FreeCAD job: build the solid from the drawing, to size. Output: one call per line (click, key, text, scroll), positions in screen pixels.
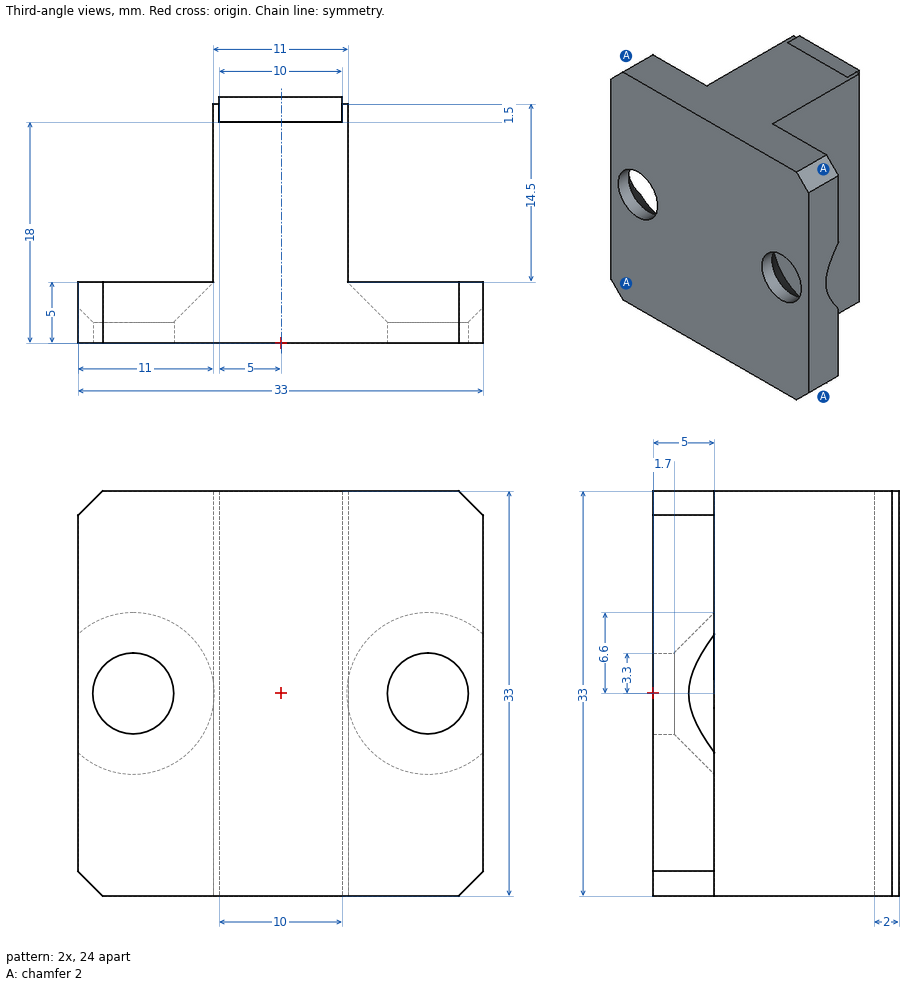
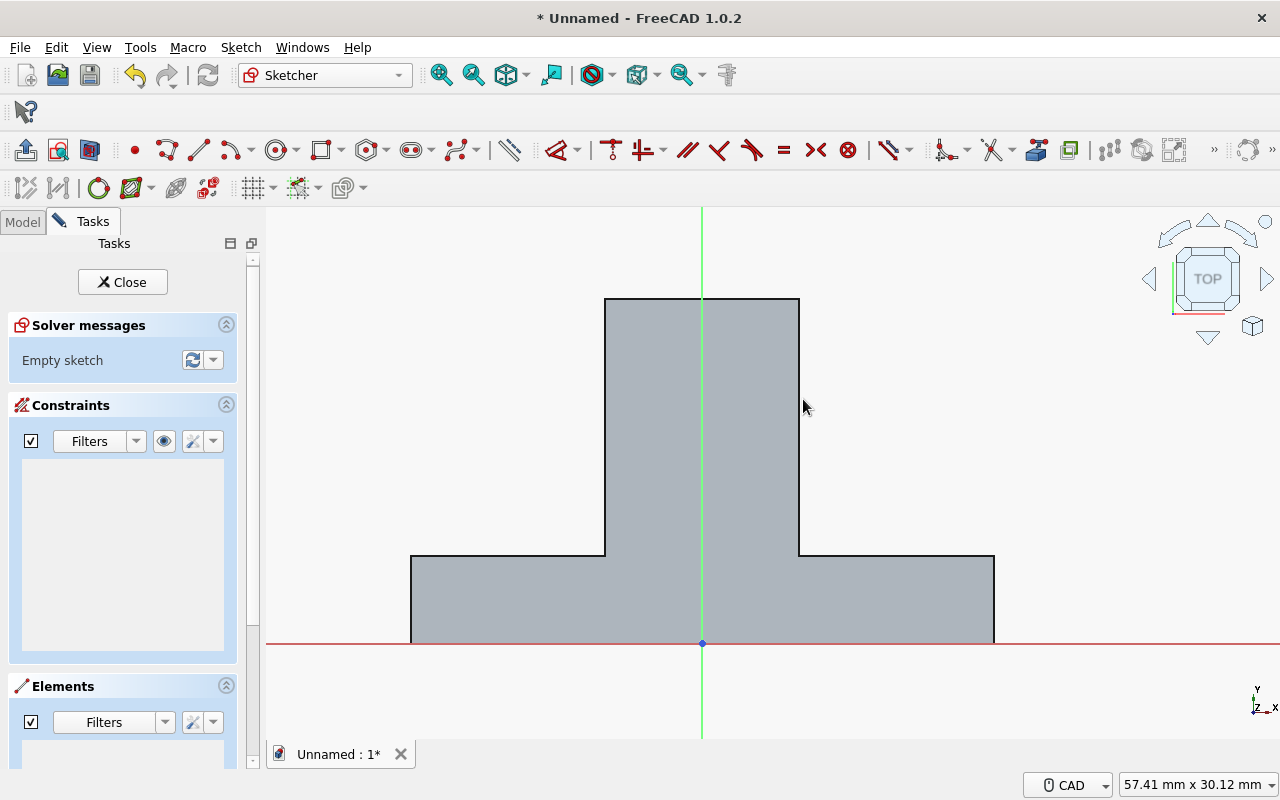
key(g)
key(r)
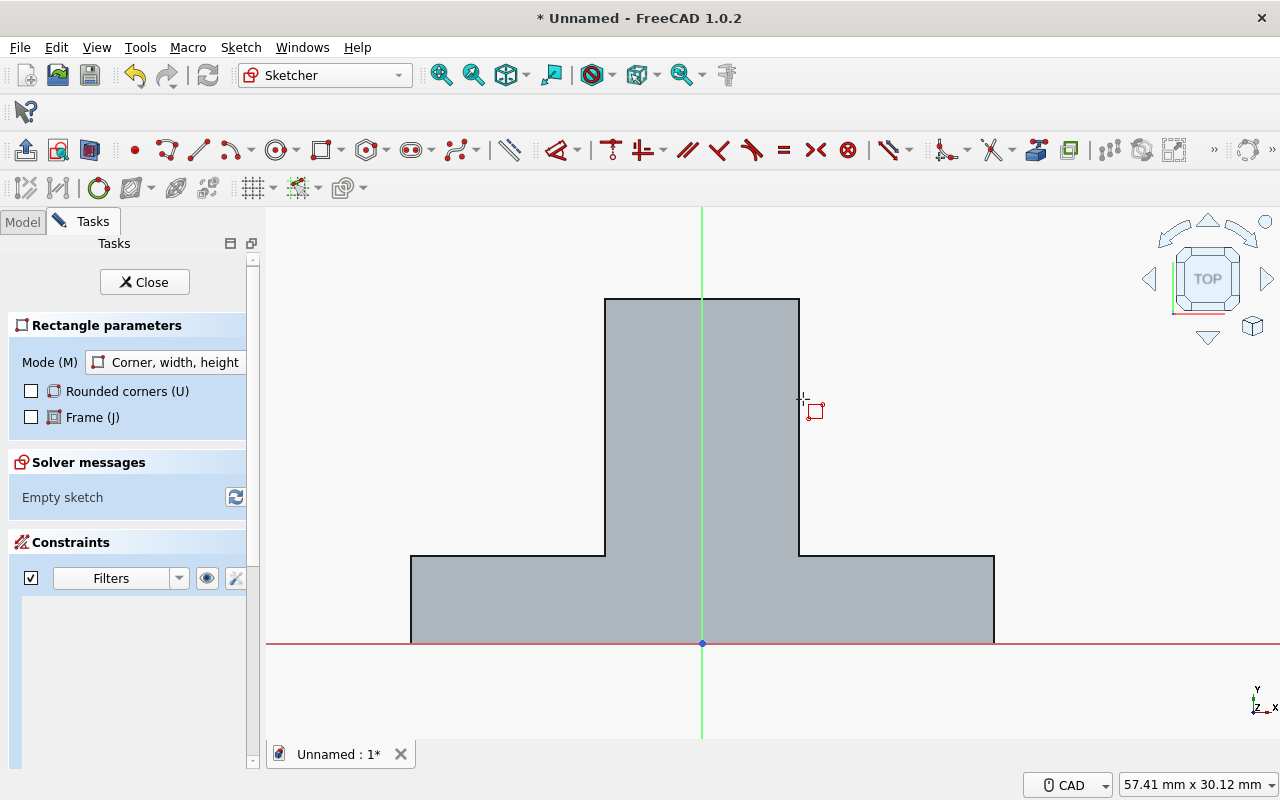
click(614, 299)
move(790, 326)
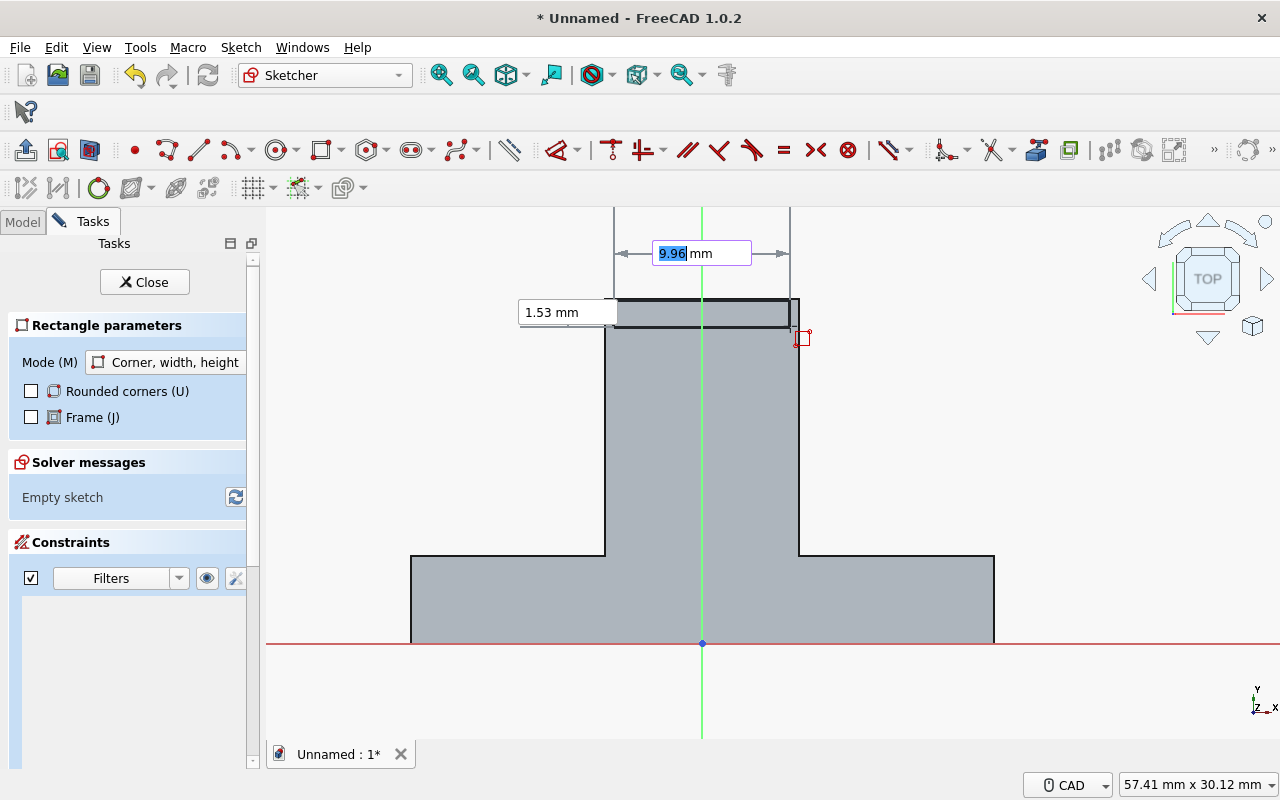
text(10)
key(Tab)
text(1.5)
key(Return)
key(Escape)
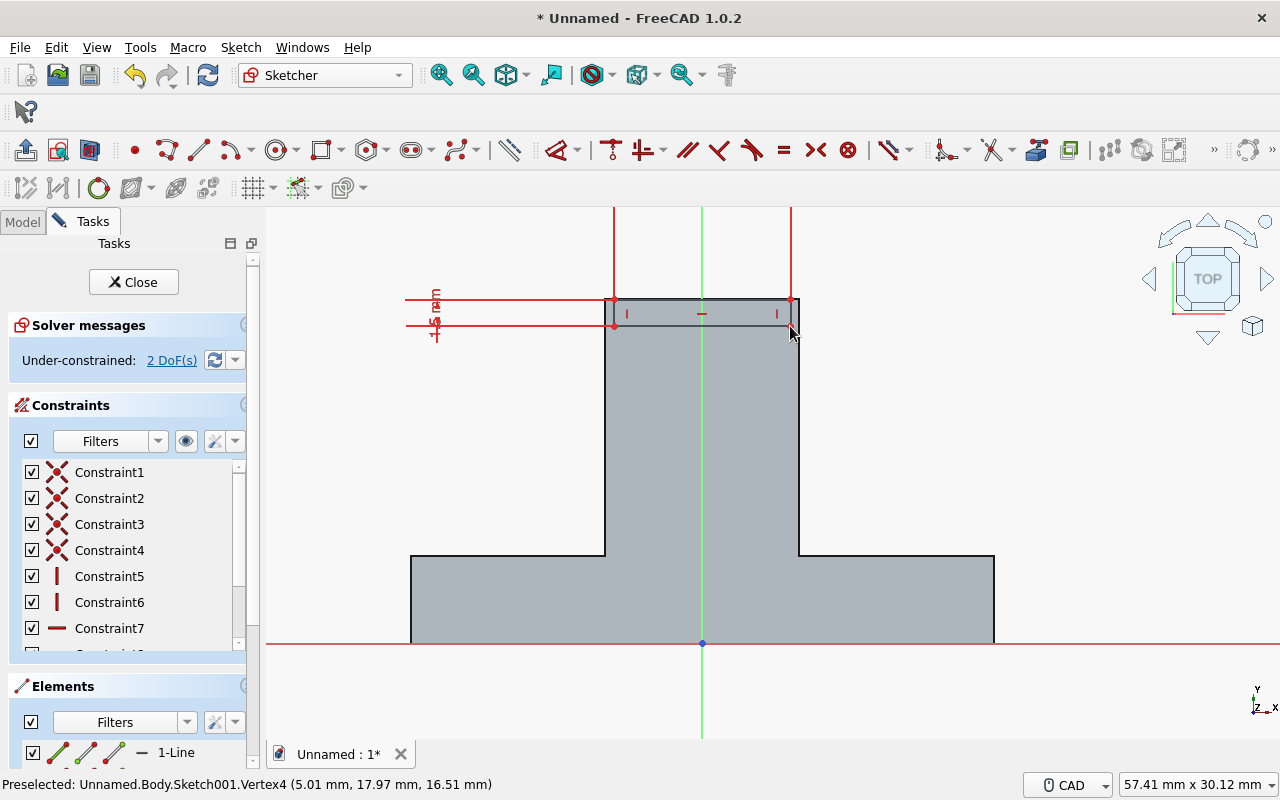
click(556, 150)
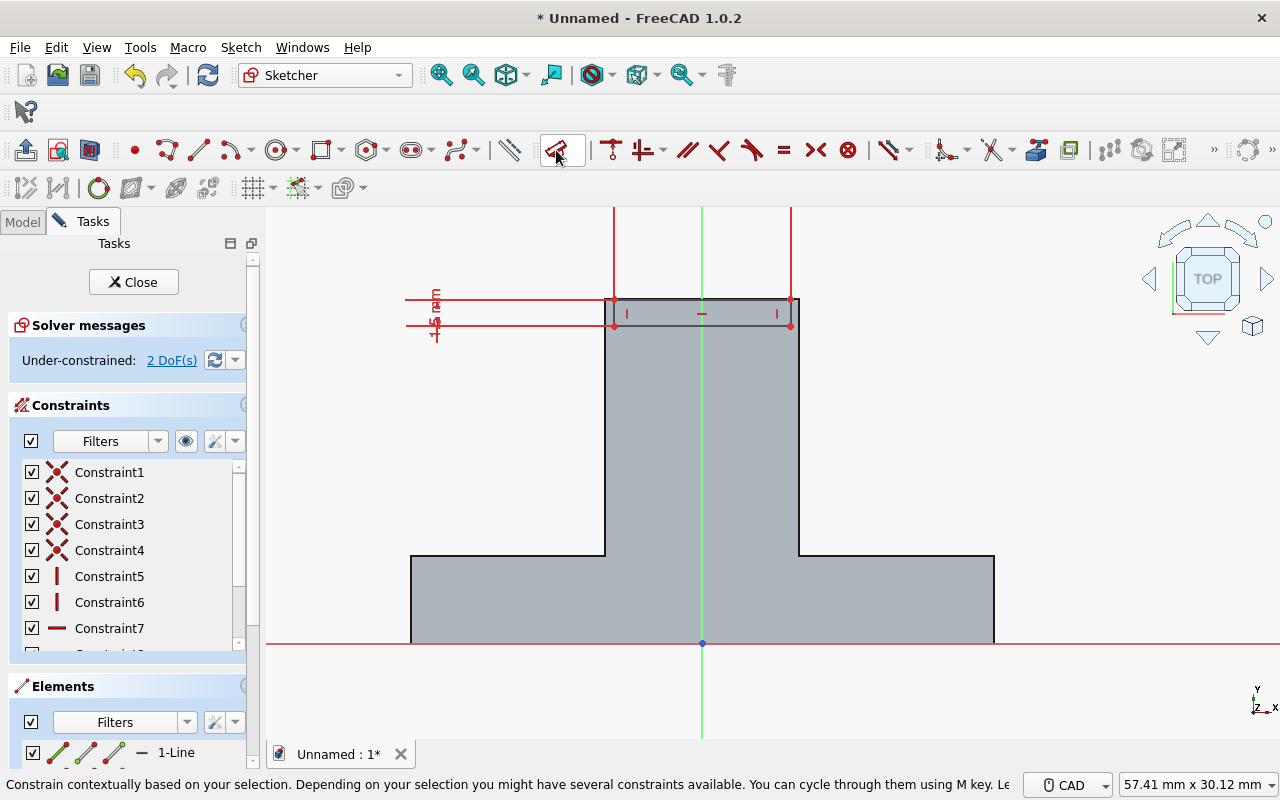
click(614, 300)
click(658, 678)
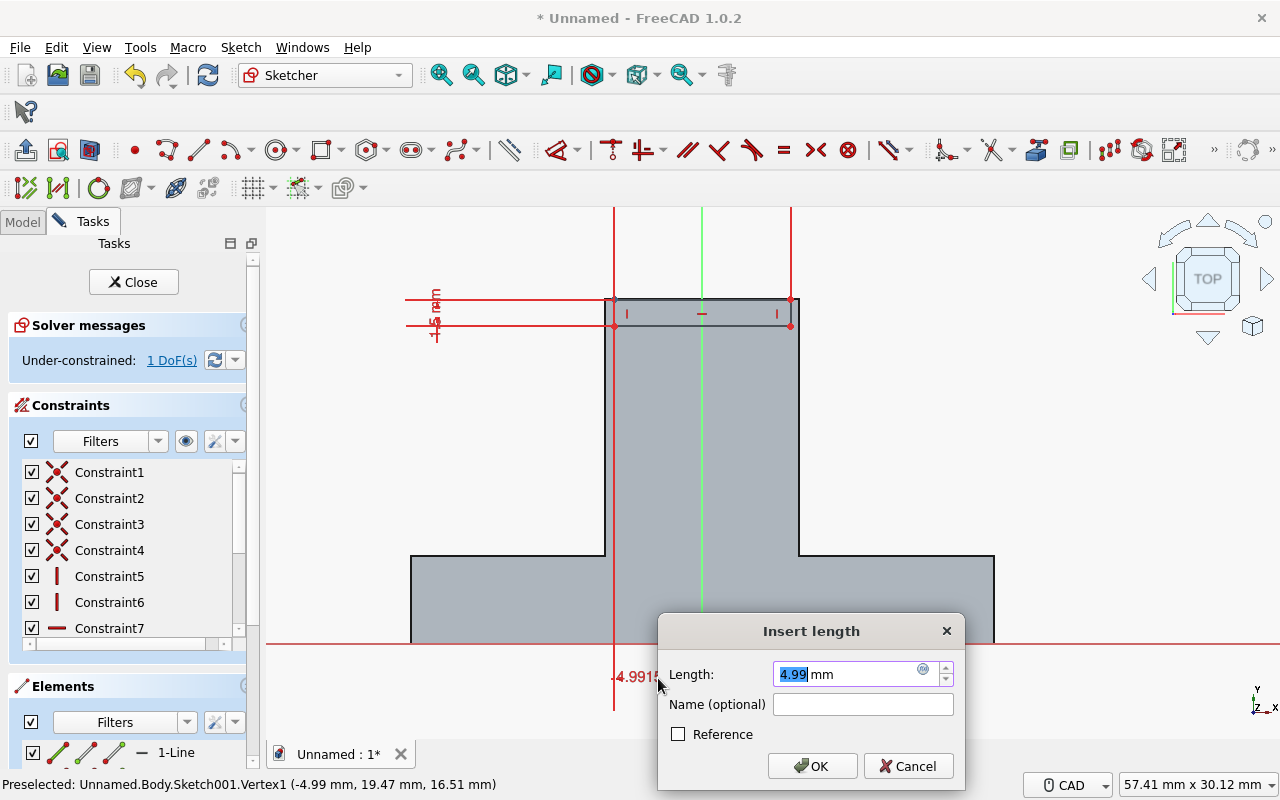
text(5)
key(Return)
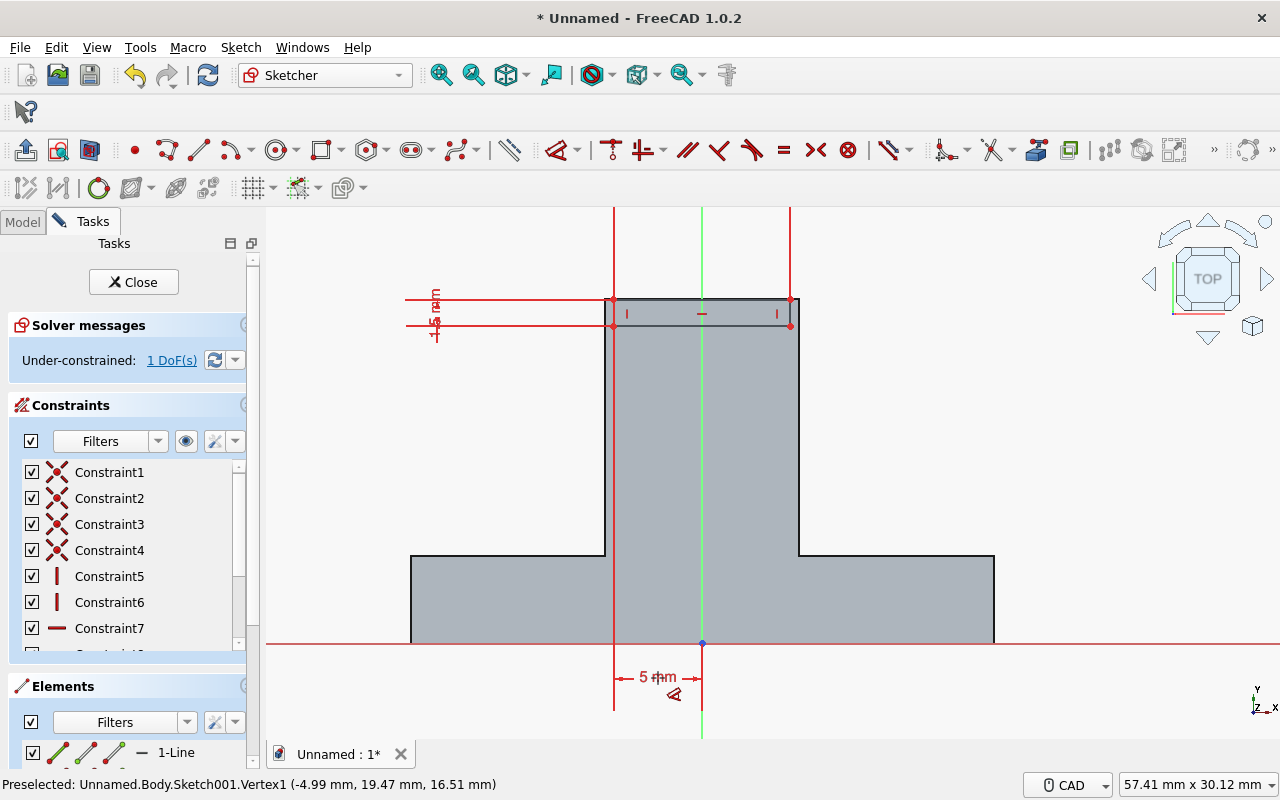
click(614, 326)
click(580, 485)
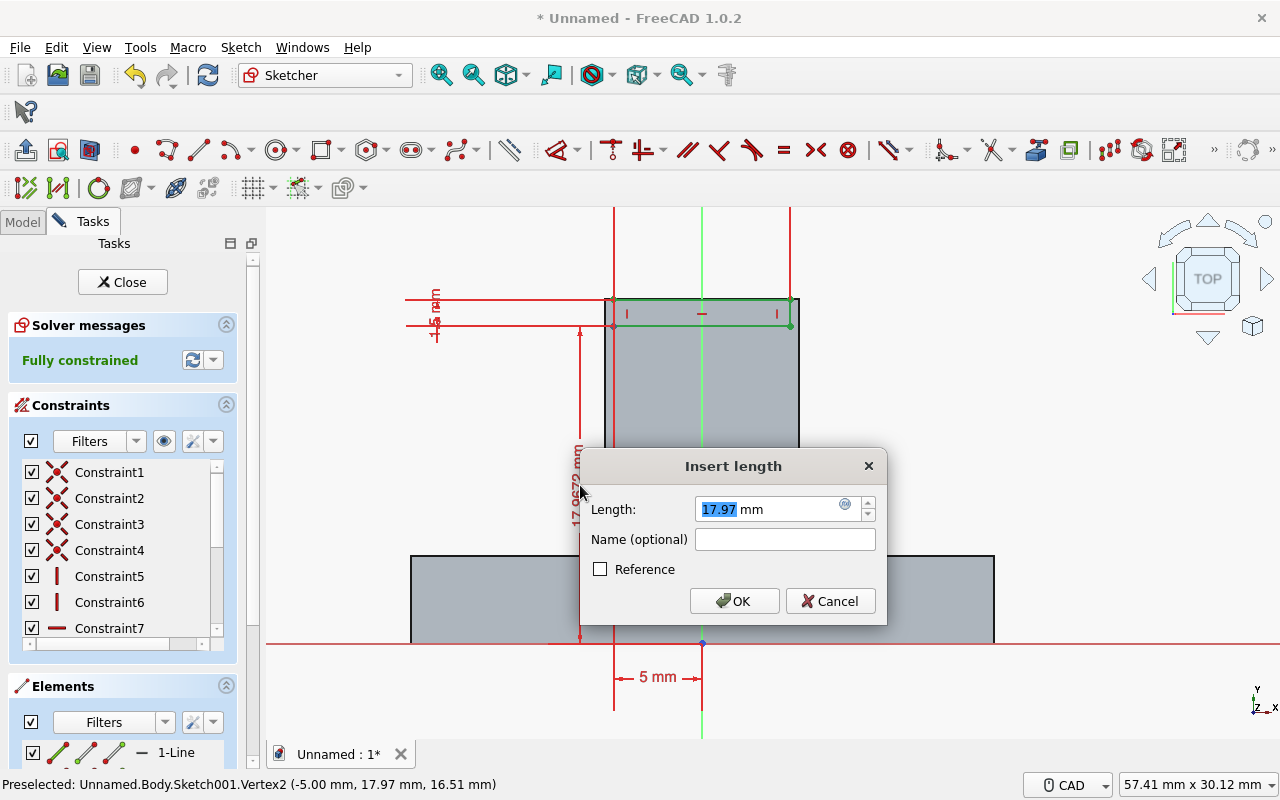
text(18)
key(Return)
key(Escape)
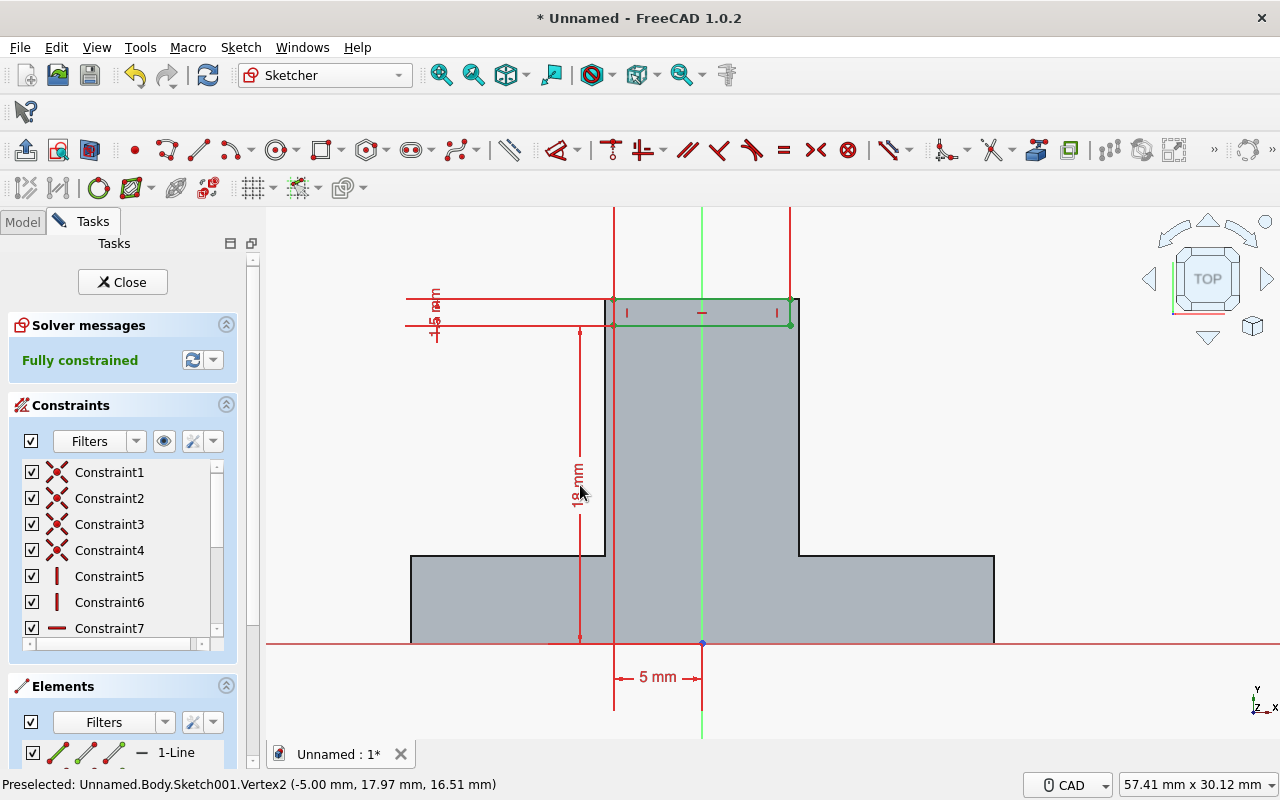
click(123, 282)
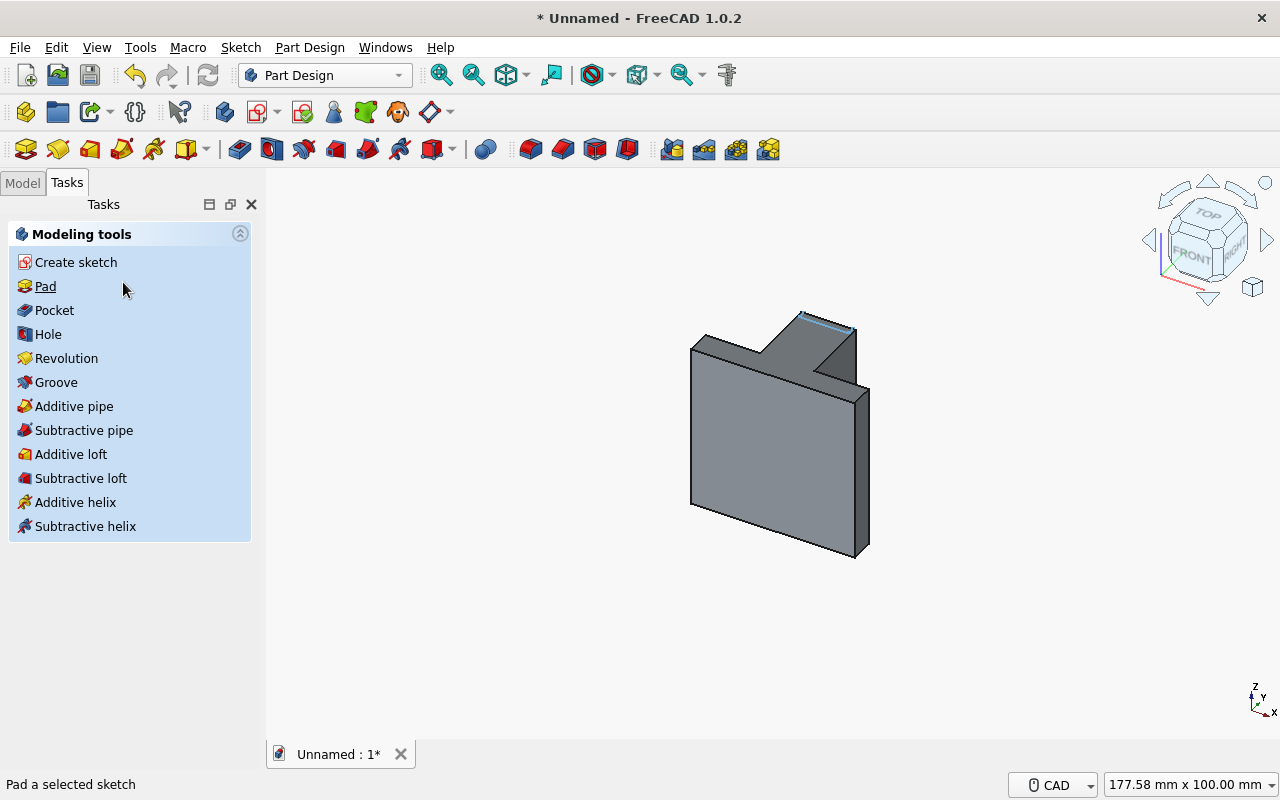
click(240, 150)